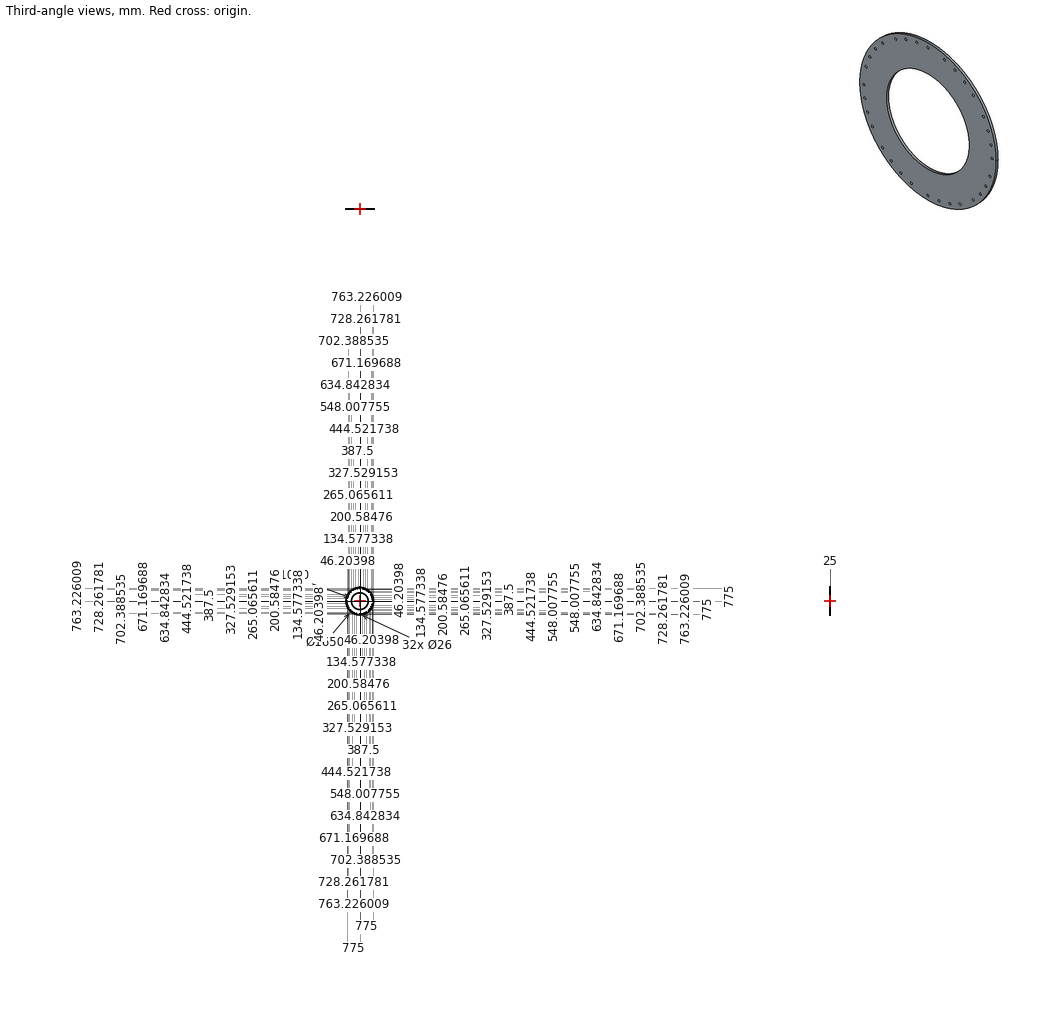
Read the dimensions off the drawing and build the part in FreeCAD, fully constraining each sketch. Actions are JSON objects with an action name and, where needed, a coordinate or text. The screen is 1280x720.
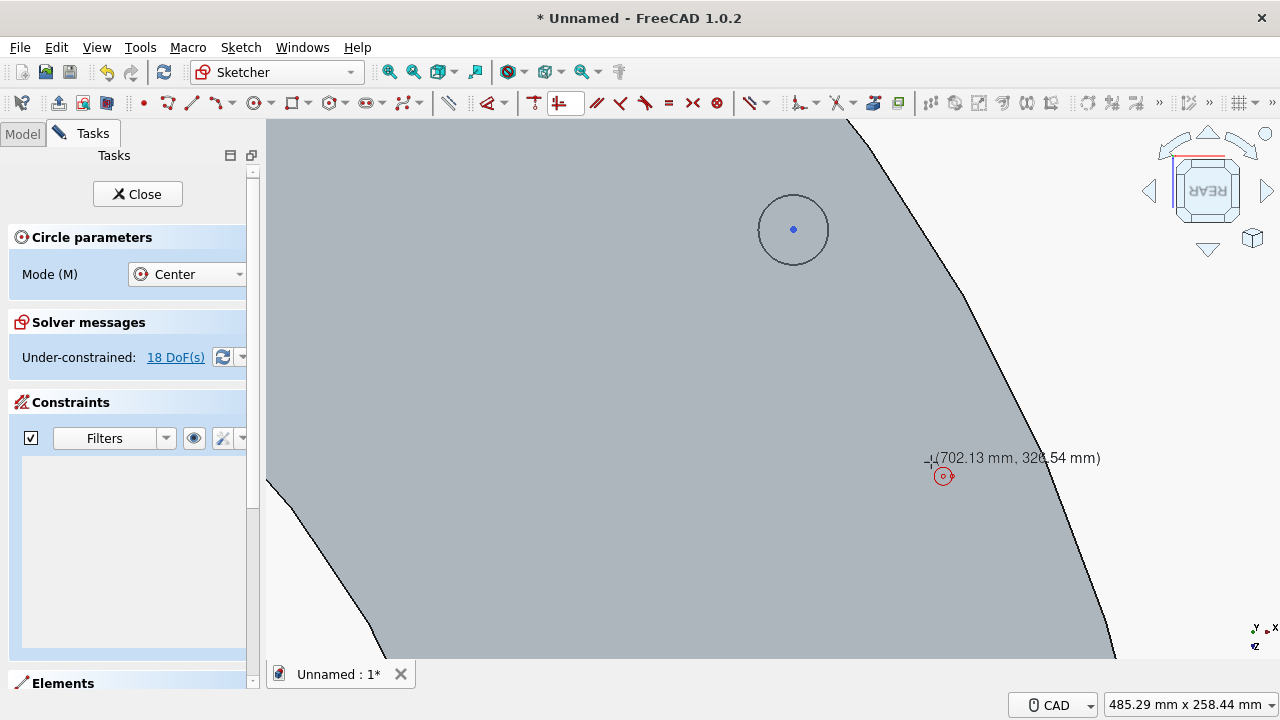
{"action": "scroll", "coordinate": [859, 295], "scroll_direction": "down", "scroll_amount": 11}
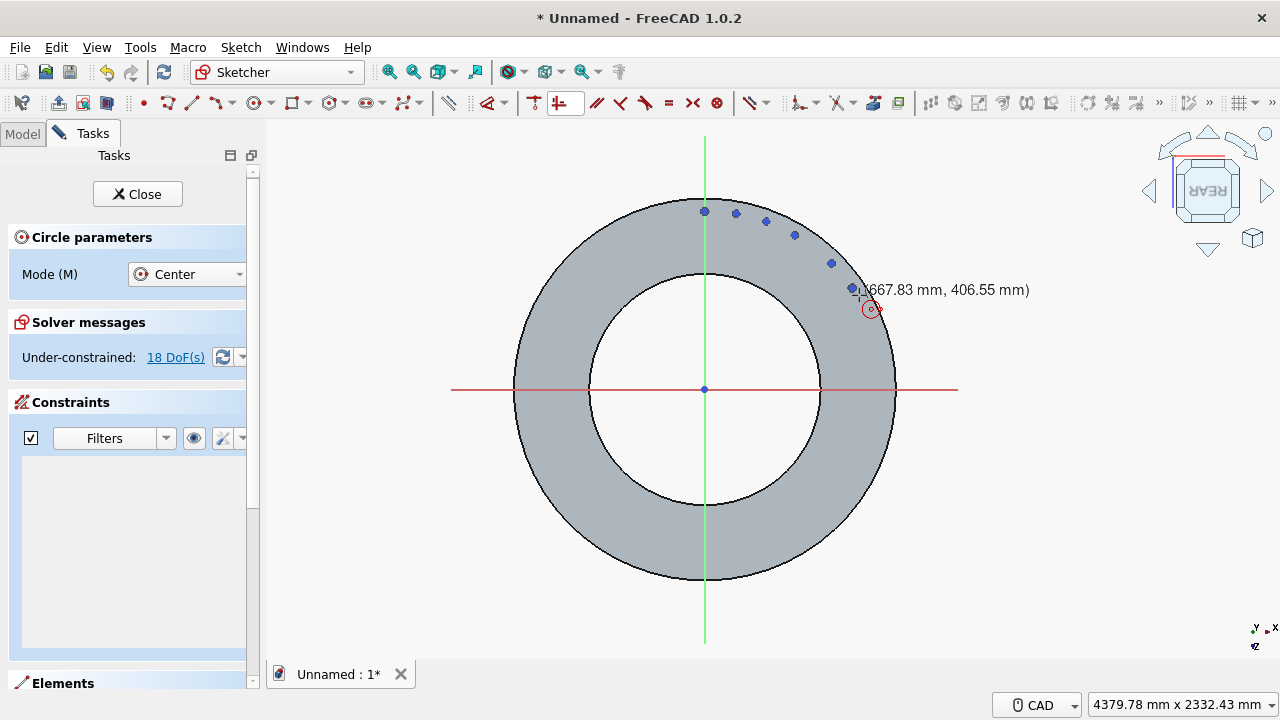
{"action": "left_click", "coordinate": [868, 314]}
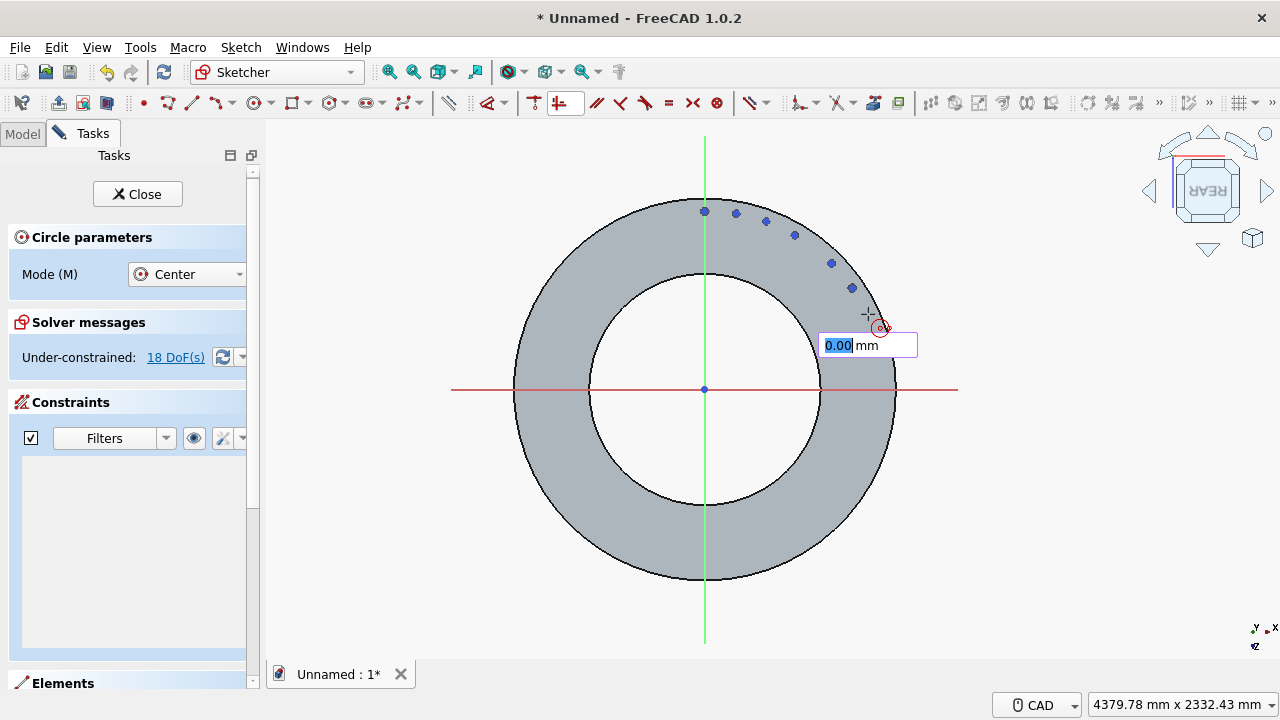
{"action": "scroll", "coordinate": [870, 312], "scroll_direction": "up", "scroll_amount": 9}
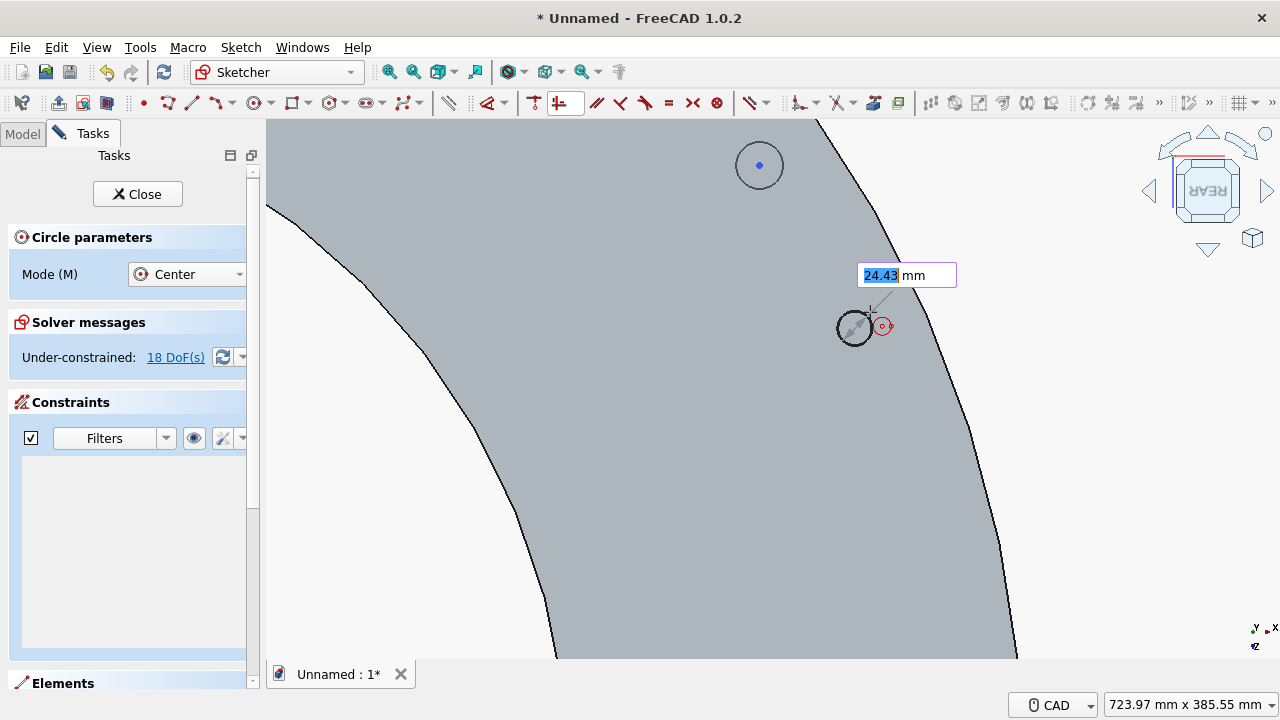
{"action": "left_click", "coordinate": [865, 308]}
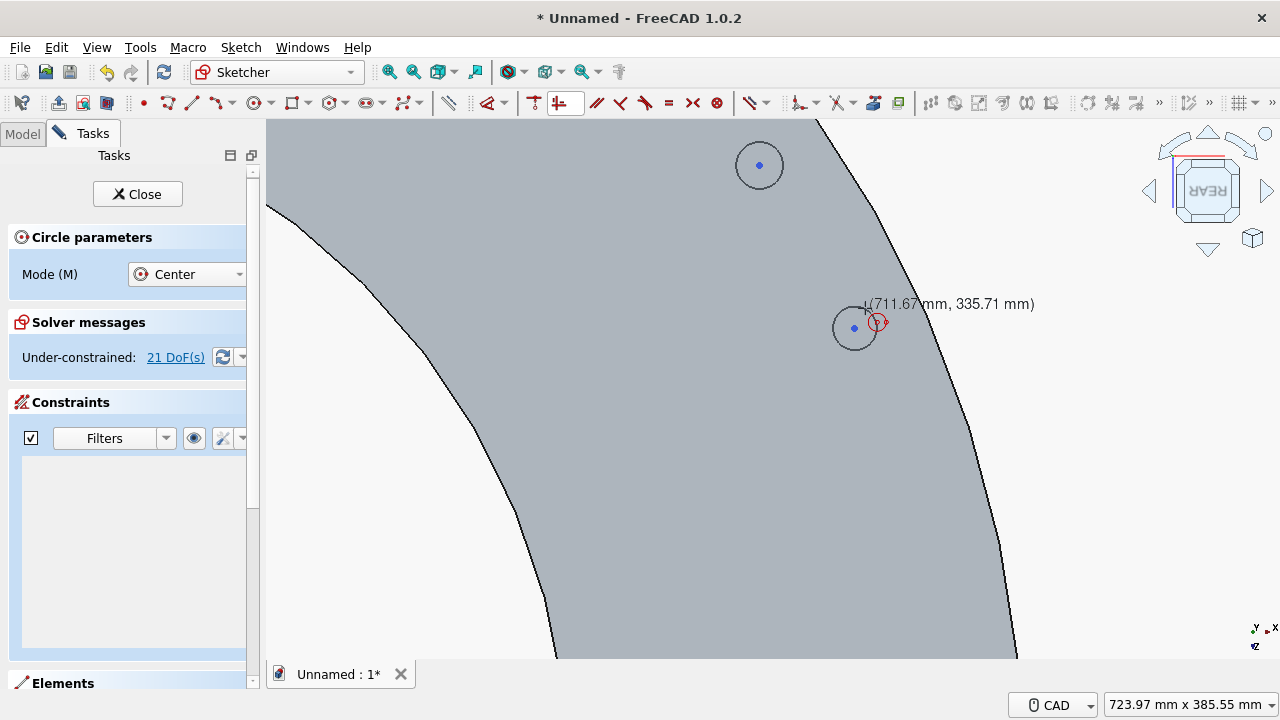
{"action": "scroll", "coordinate": [917, 498], "scroll_direction": "up", "scroll_amount": 2}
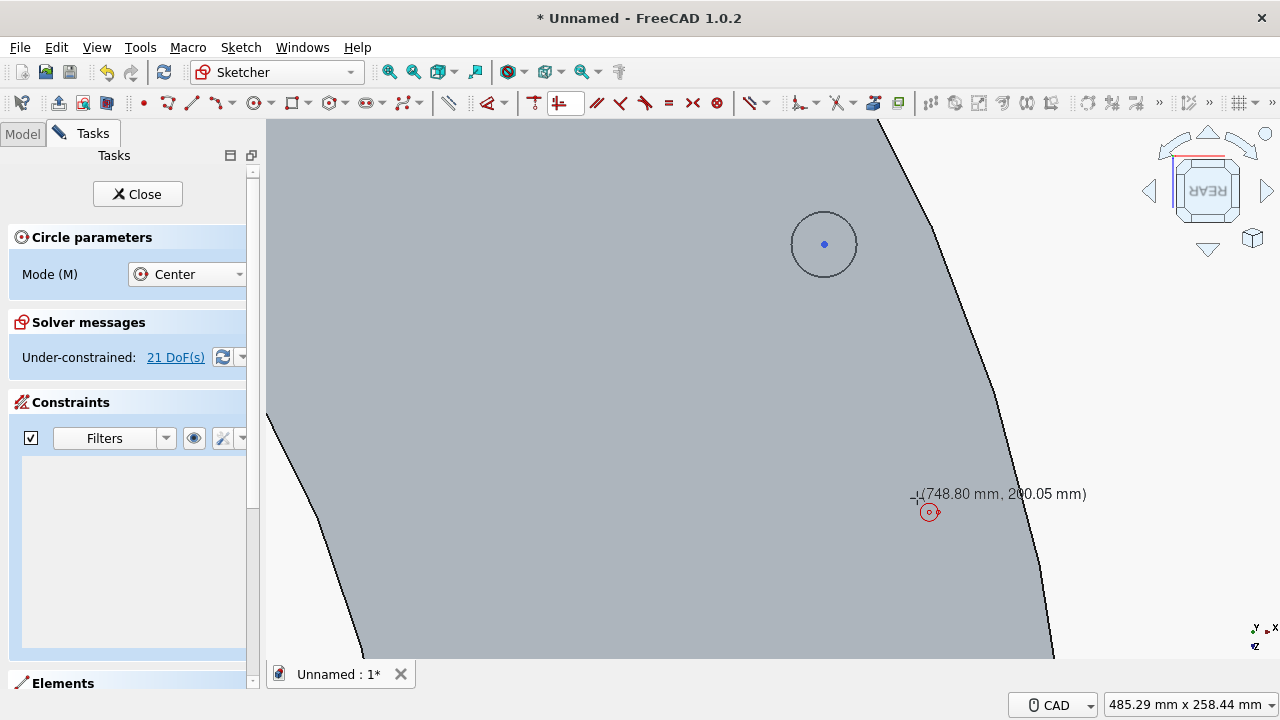
{"action": "scroll", "coordinate": [873, 323], "scroll_direction": "down", "scroll_amount": 11}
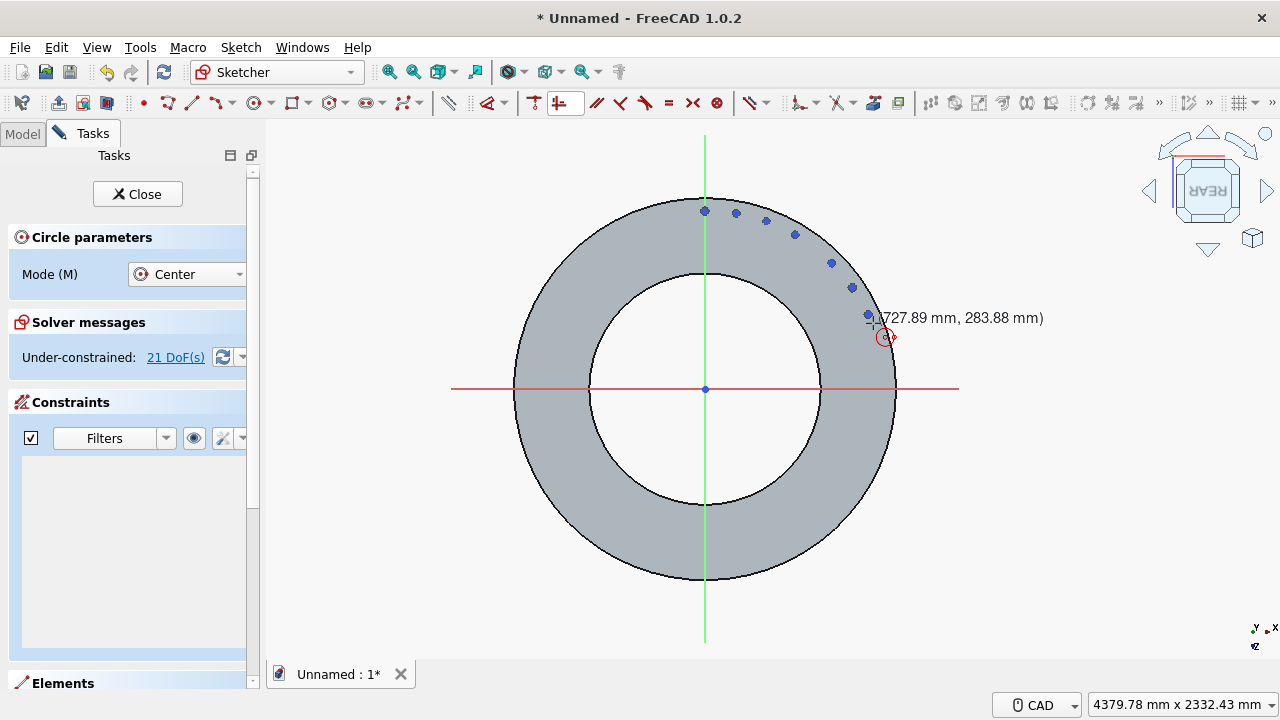
{"action": "left_click", "coordinate": [878, 343]}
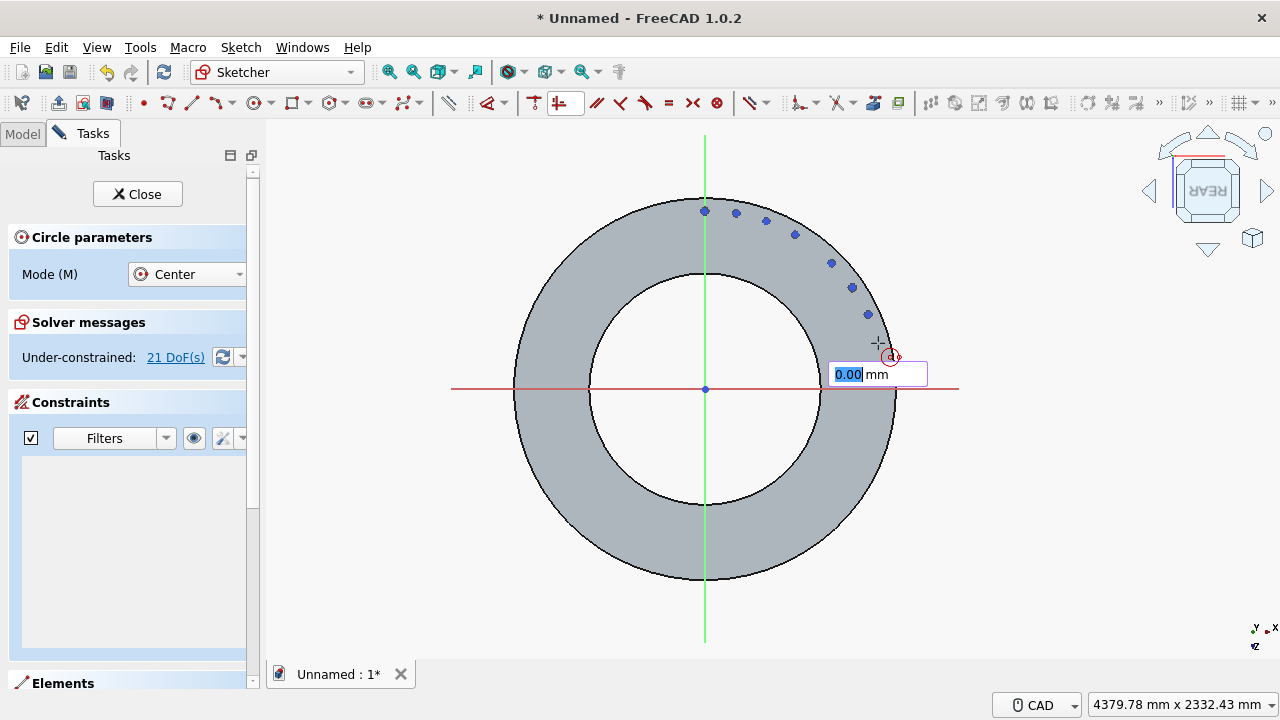
{"action": "scroll", "coordinate": [880, 341], "scroll_direction": "up", "scroll_amount": 9}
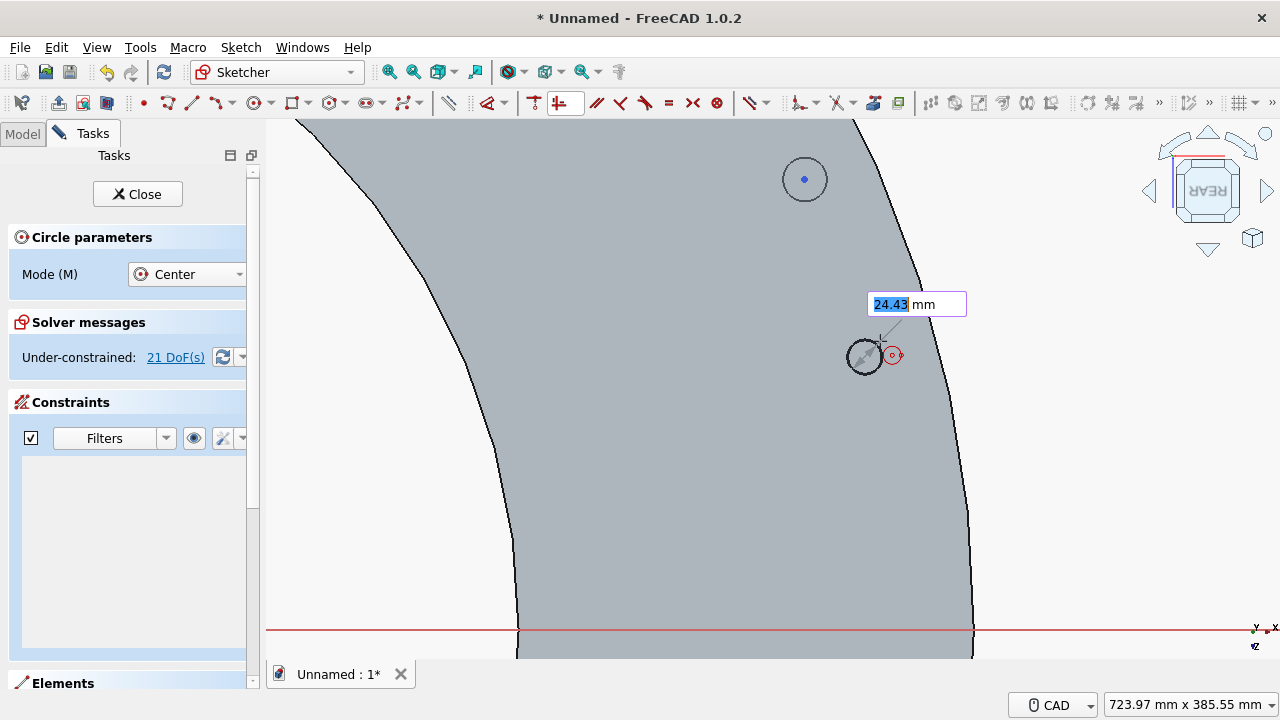
{"action": "left_click", "coordinate": [880, 337]}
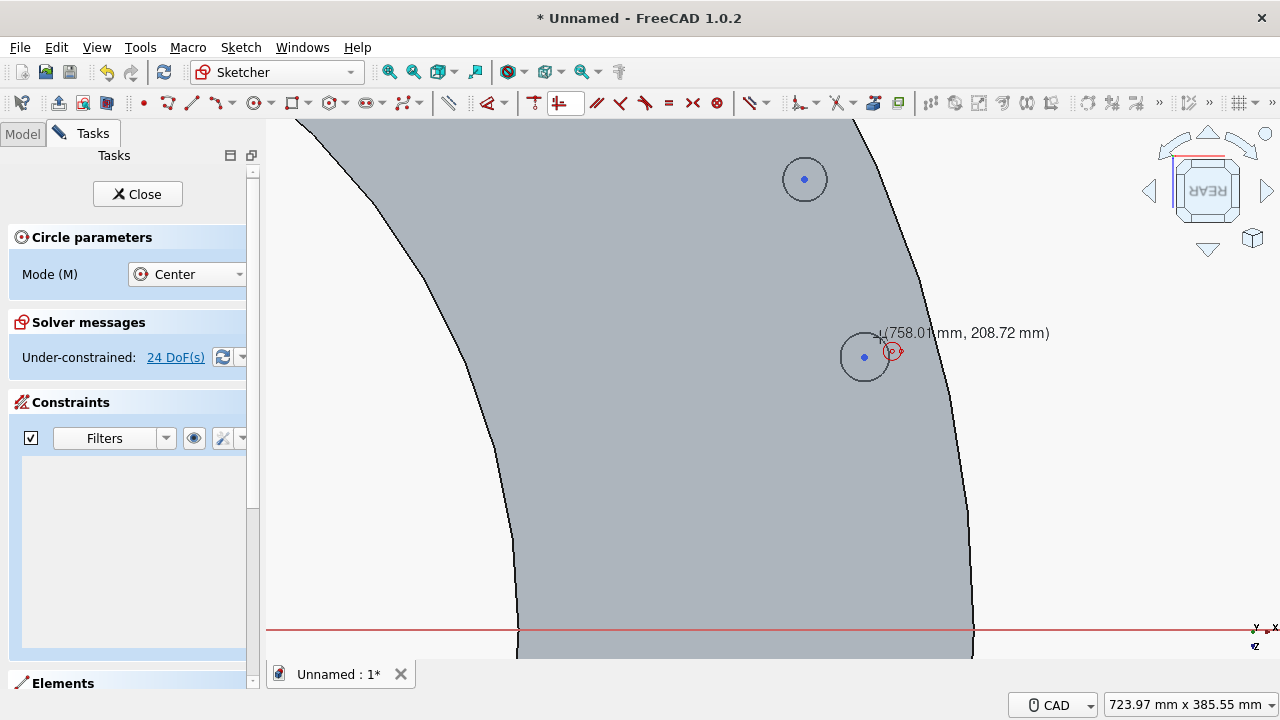
{"action": "scroll", "coordinate": [904, 630], "scroll_direction": "up", "scroll_amount": 2}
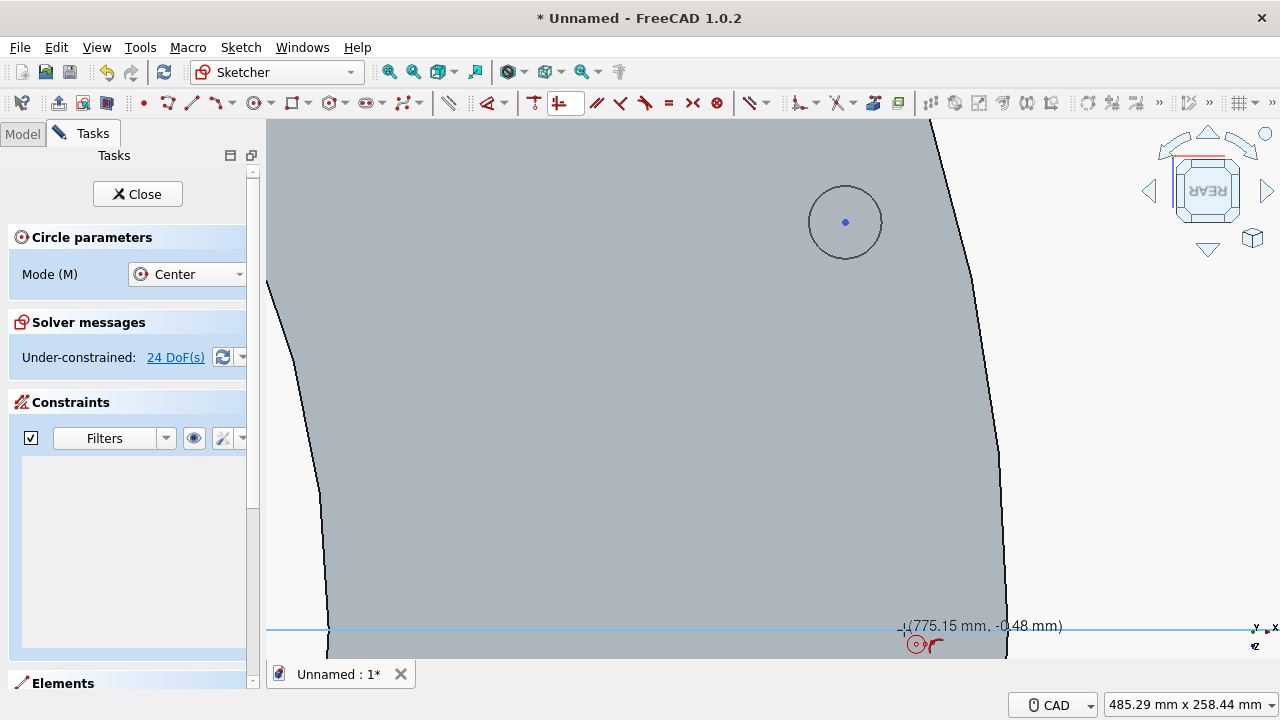
{"action": "scroll", "coordinate": [882, 359], "scroll_direction": "down", "scroll_amount": 11}